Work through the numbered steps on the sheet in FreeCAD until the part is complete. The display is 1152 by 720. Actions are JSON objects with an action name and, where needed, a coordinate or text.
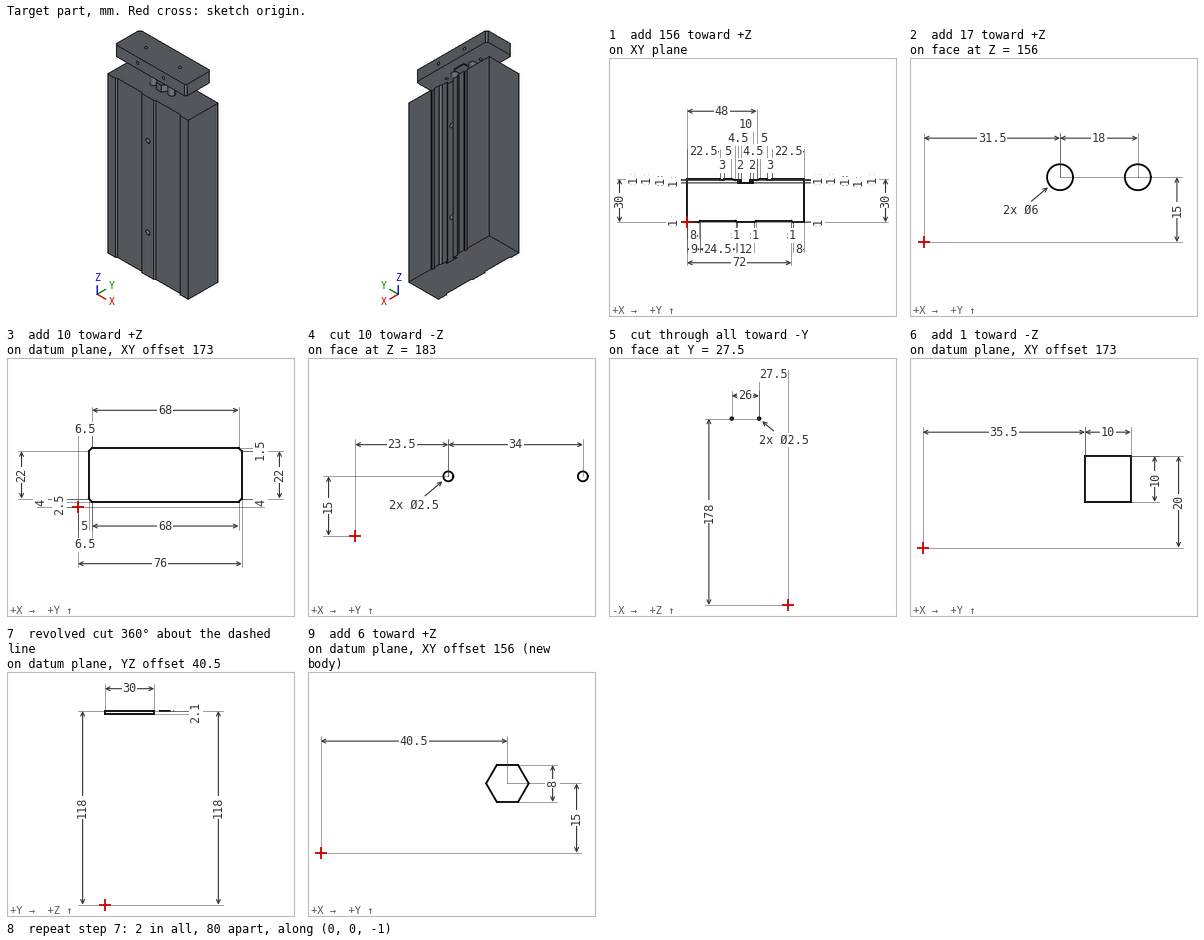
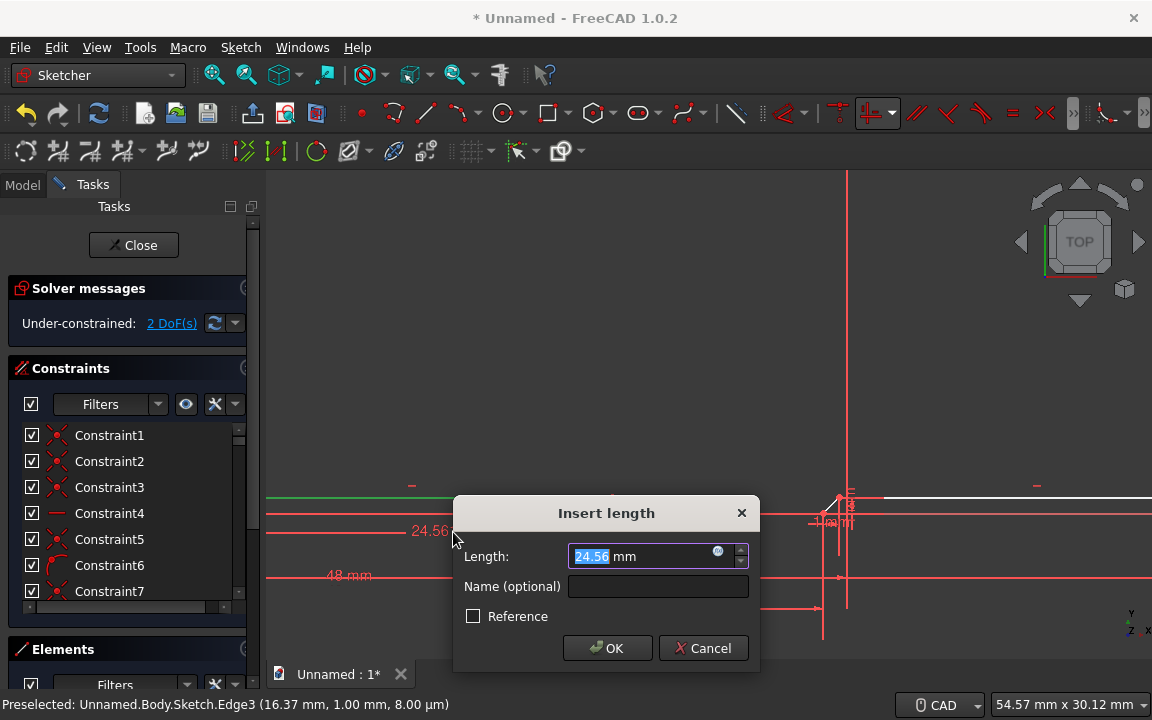
{"action": "type", "text": "24.5"}
{"action": "key", "text": "Return"}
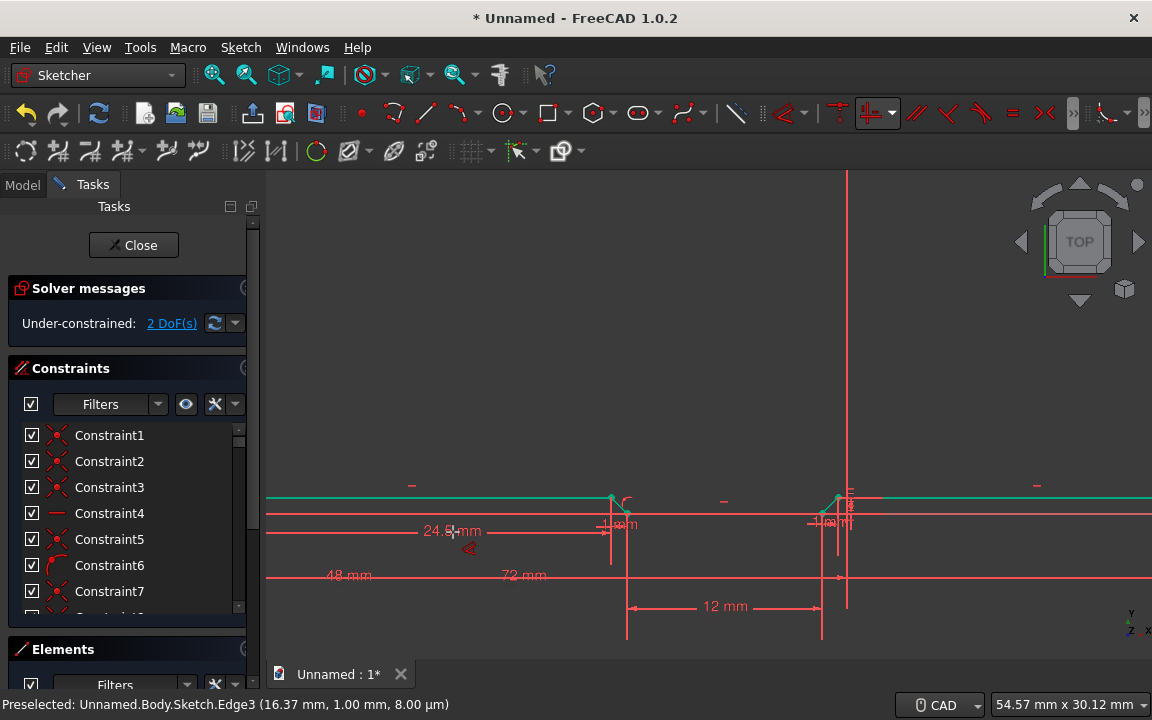
{"action": "scroll", "coordinate": [591, 498], "scroll_direction": "down", "scroll_amount": 5}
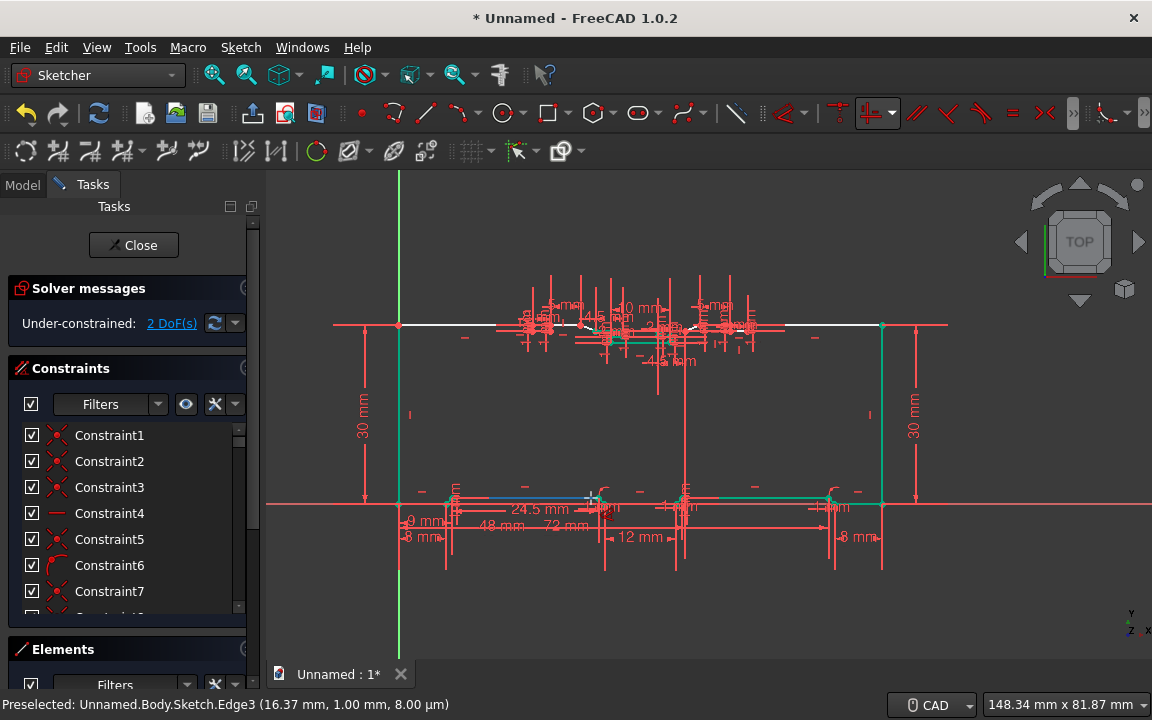
{"action": "left_click", "coordinate": [842, 325]}
{"action": "left_click", "coordinate": [815, 291]}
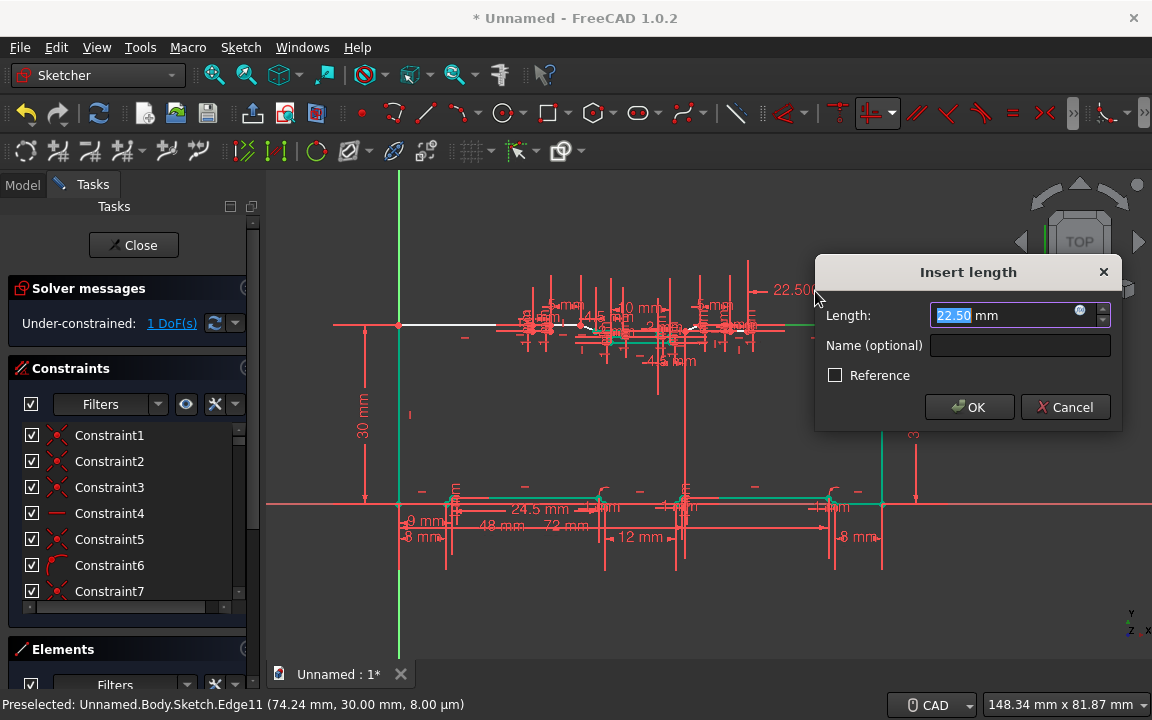
{"action": "type", "text": "22.5"}
{"action": "key", "text": "Return"}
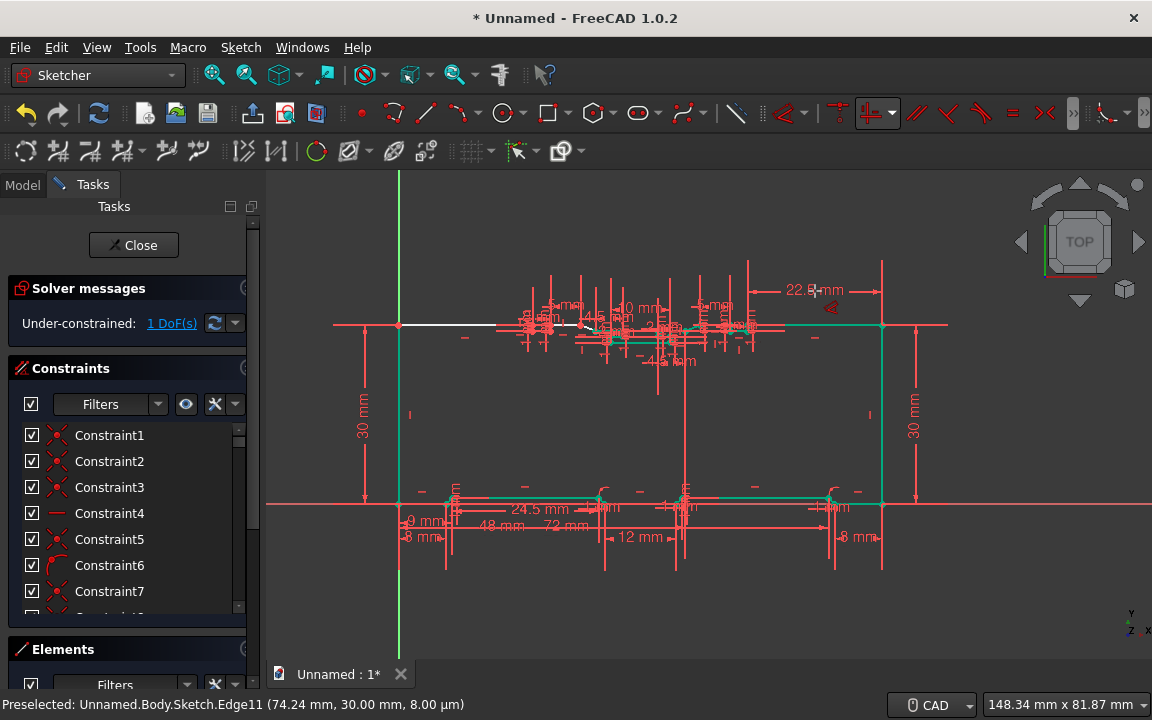
{"action": "left_click", "coordinate": [493, 325]}
{"action": "left_click", "coordinate": [466, 291]}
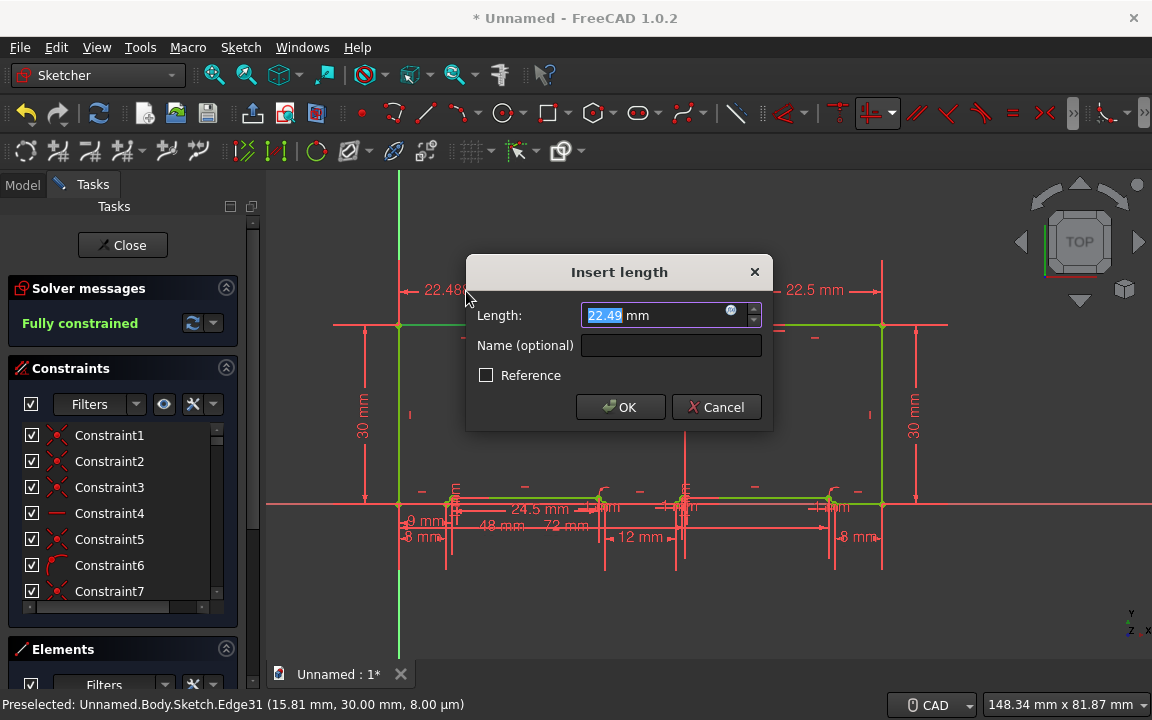
{"action": "type", "text": "22.5"}
{"action": "key", "text": "Return"}
{"action": "key", "text": "Escape"}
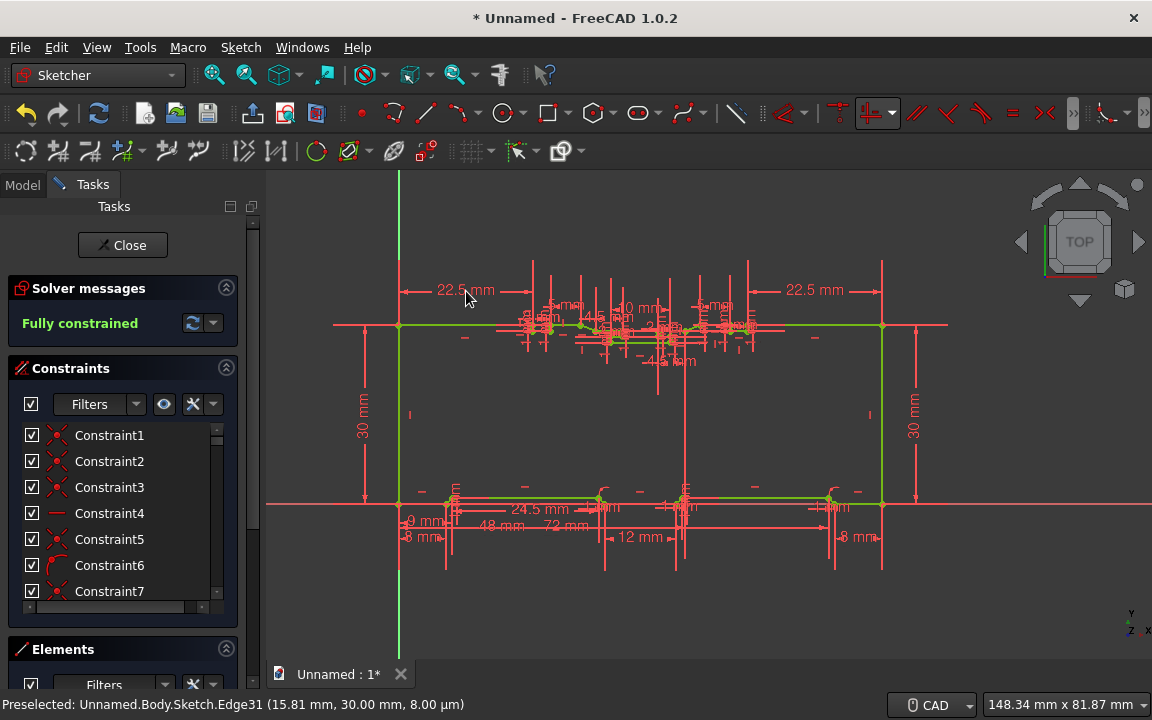
{"action": "left_click", "coordinate": [123, 245]}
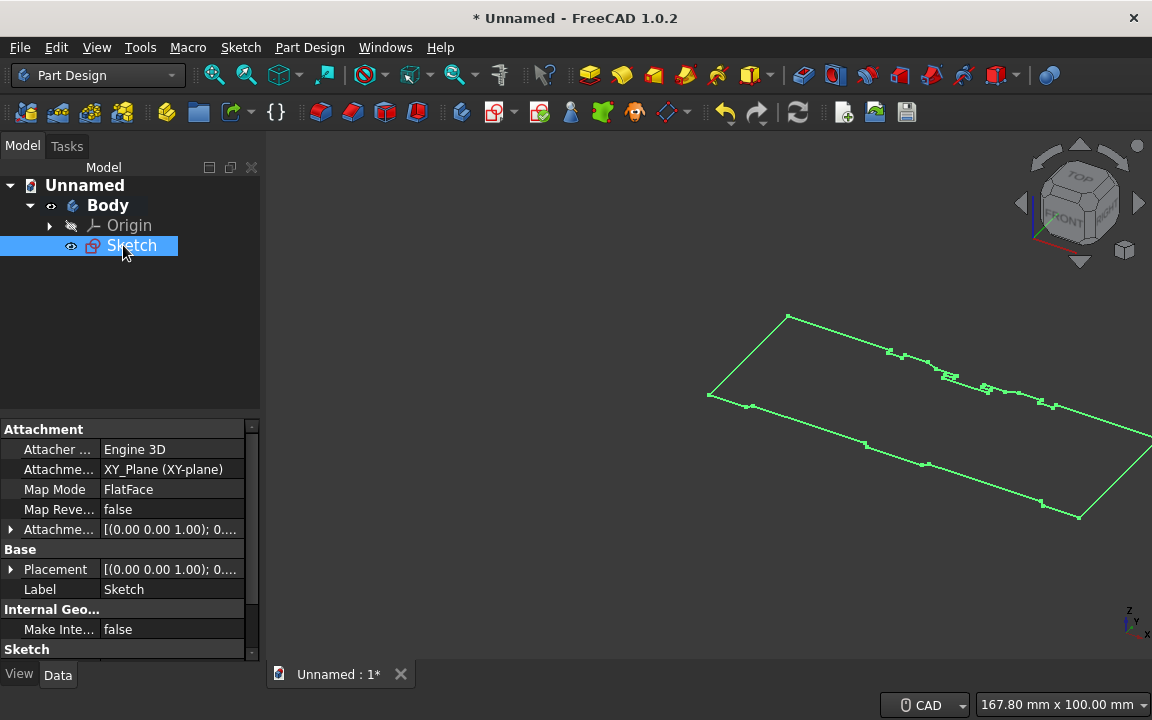
{"action": "left_click", "coordinate": [590, 76]}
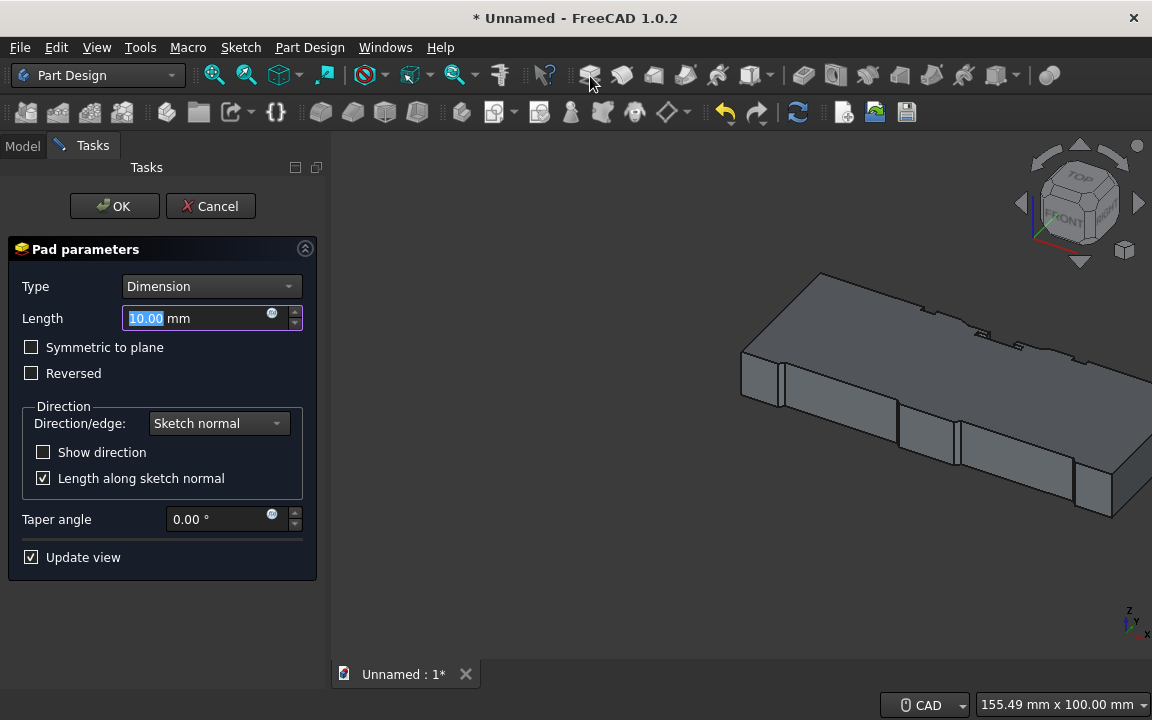
{"action": "type", "text": "156"}
{"action": "key", "text": "Tab"}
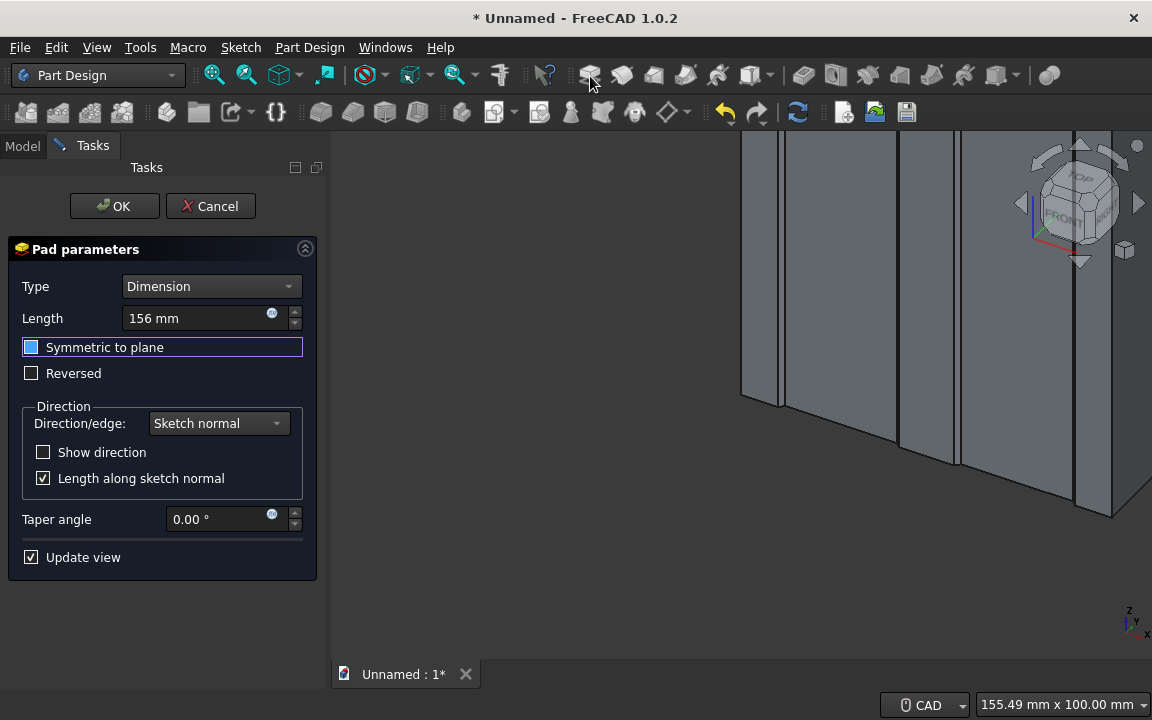
{"action": "left_click", "coordinate": [115, 206]}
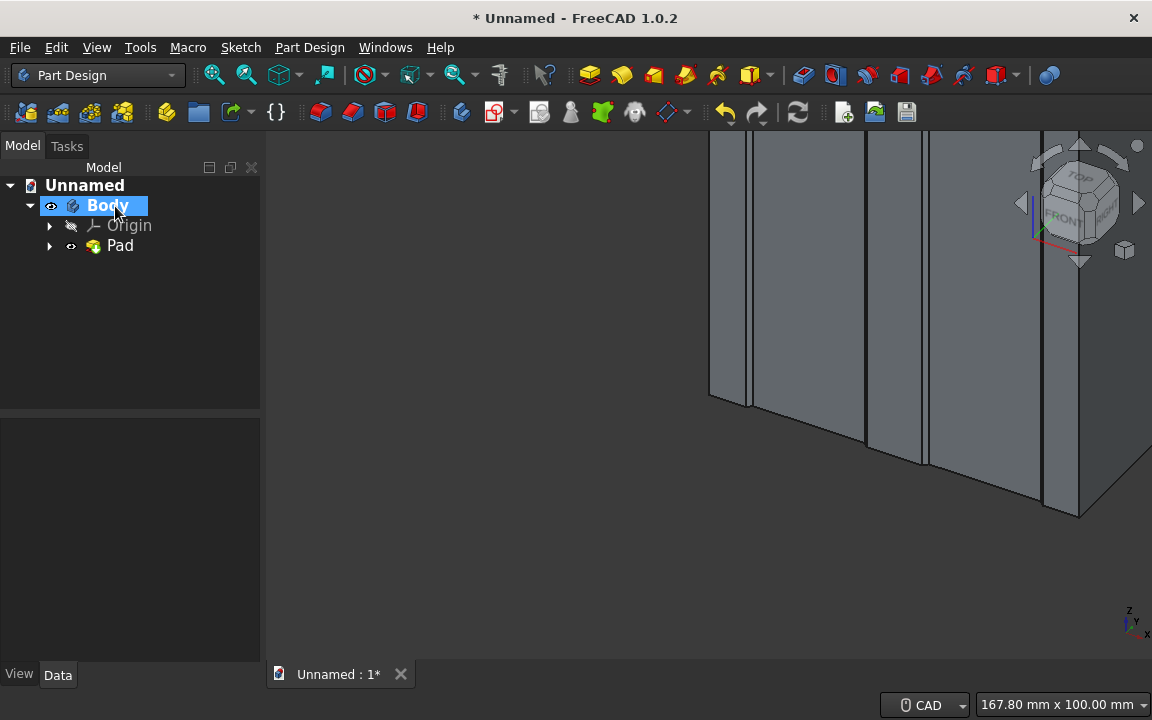
{"action": "key", "text": "v f"}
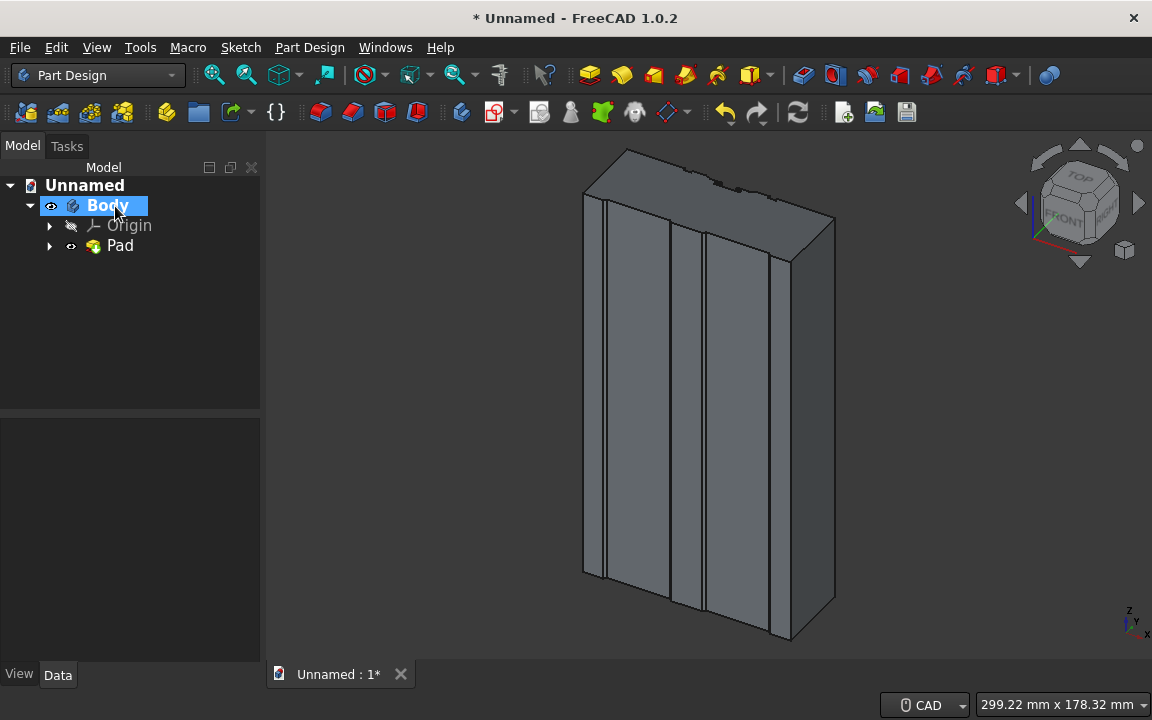
{"action": "left_click", "coordinate": [768, 224]}